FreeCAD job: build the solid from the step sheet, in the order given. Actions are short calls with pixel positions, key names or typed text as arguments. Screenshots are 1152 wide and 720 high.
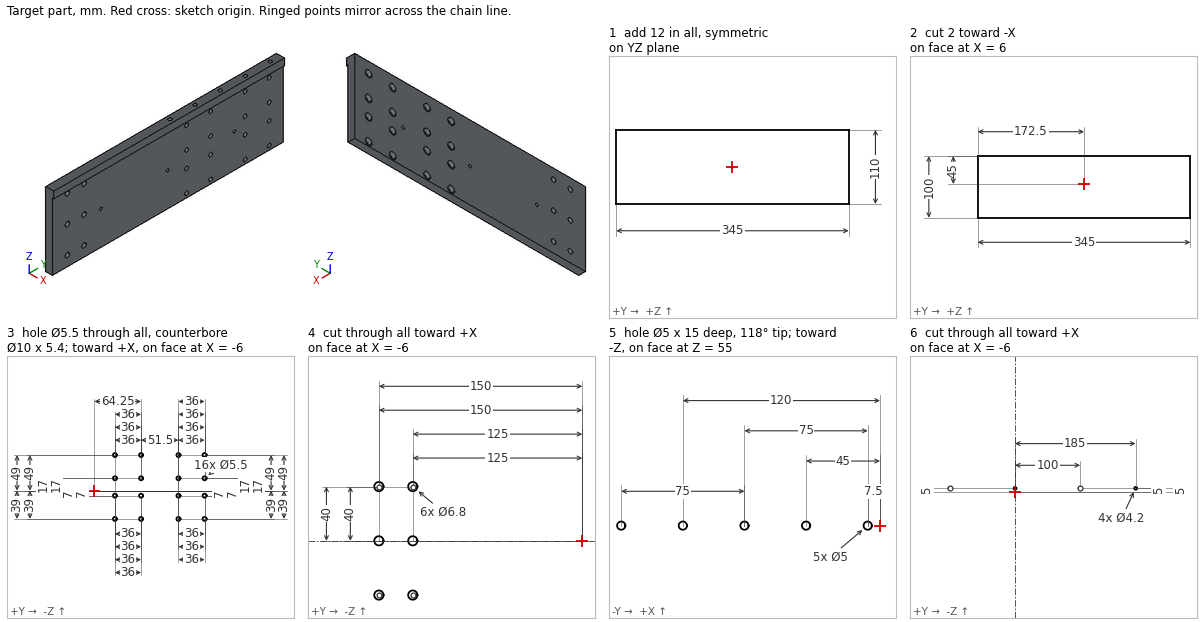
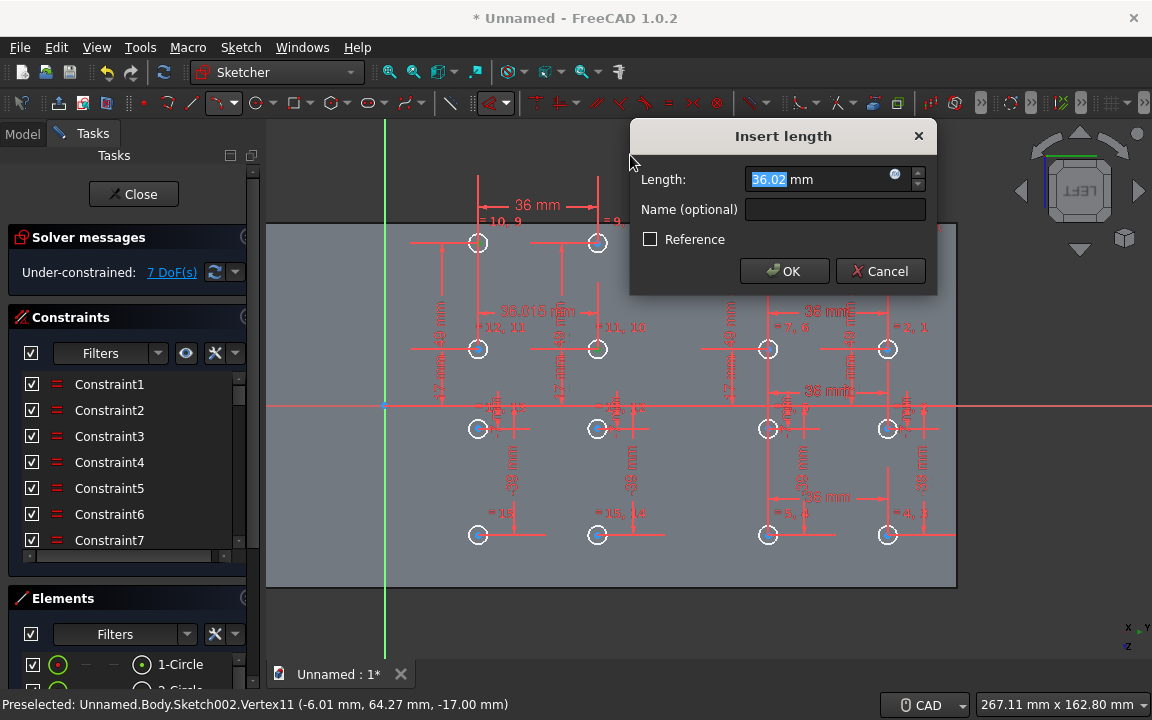
text(36)
key(Return)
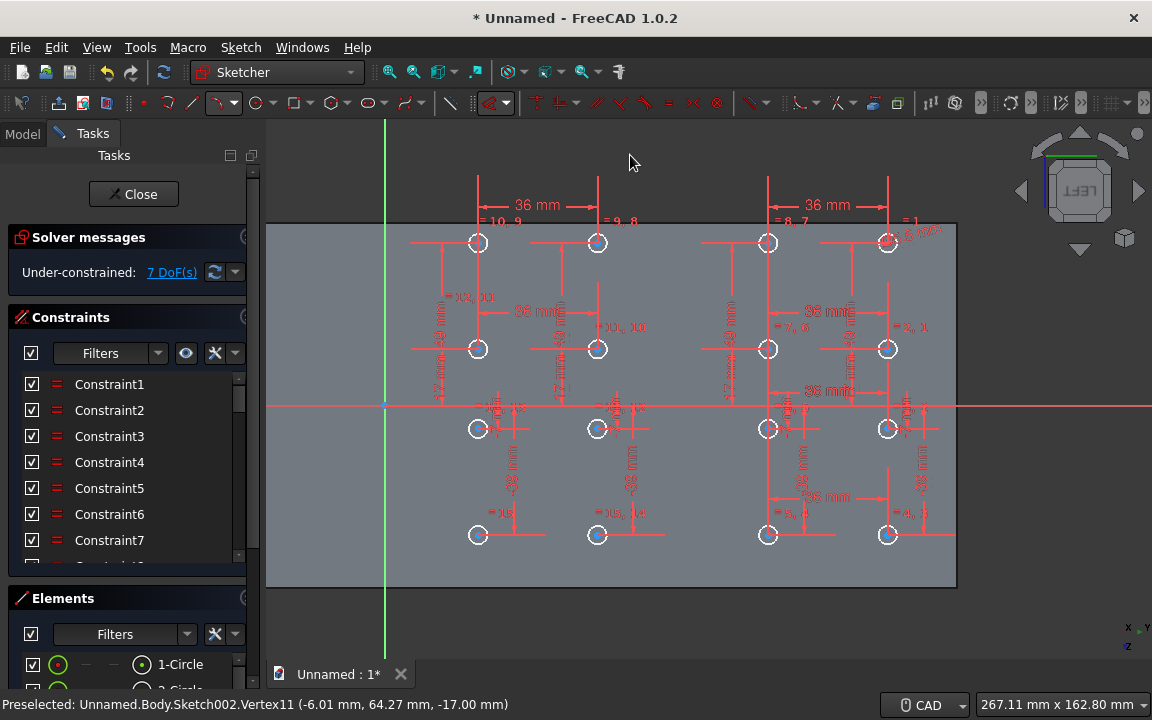
click(598, 349)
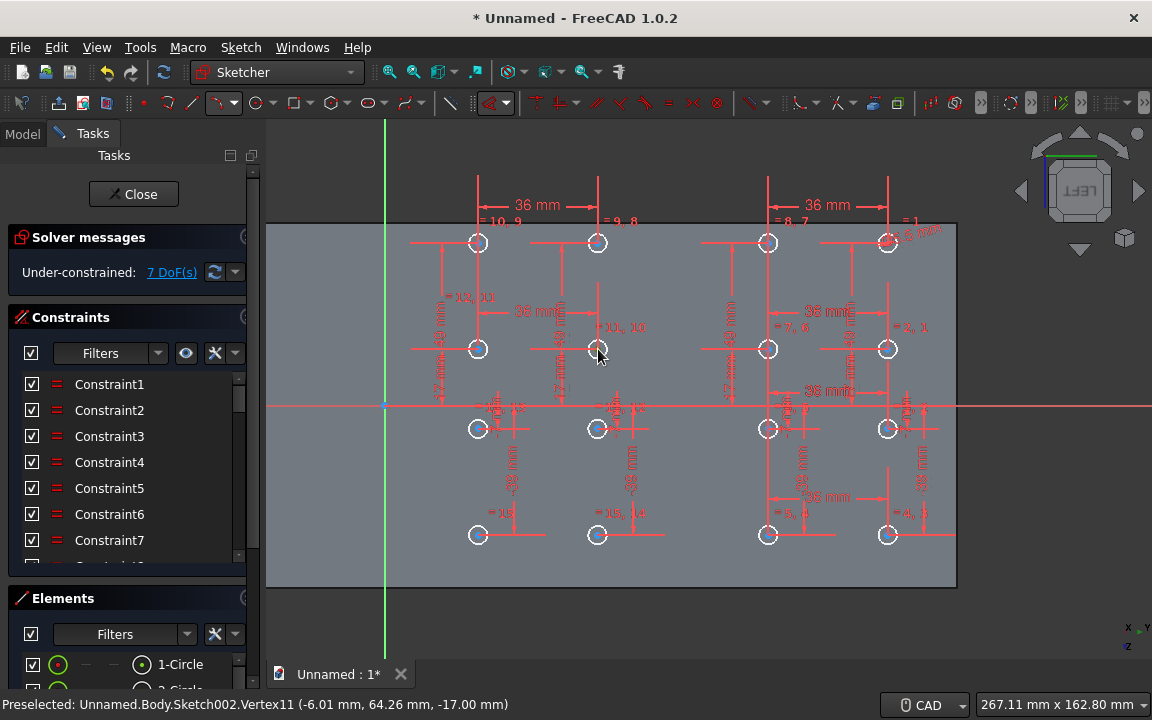
click(478, 349)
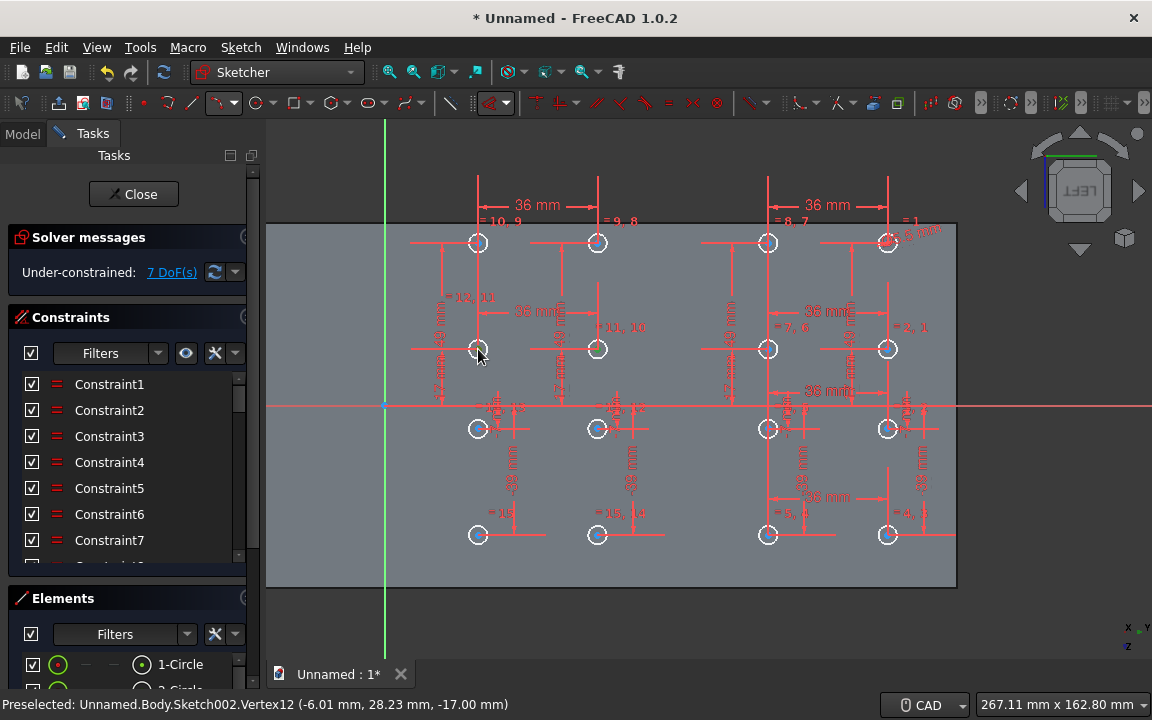
key(l)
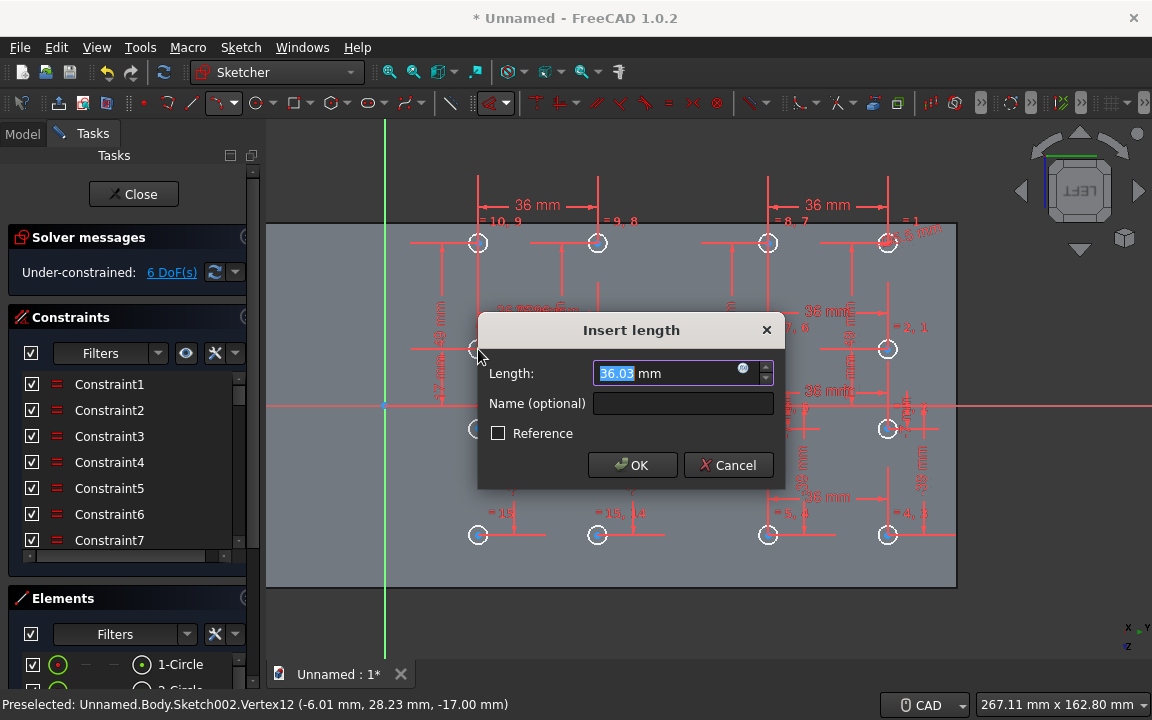
text(36)
key(Return)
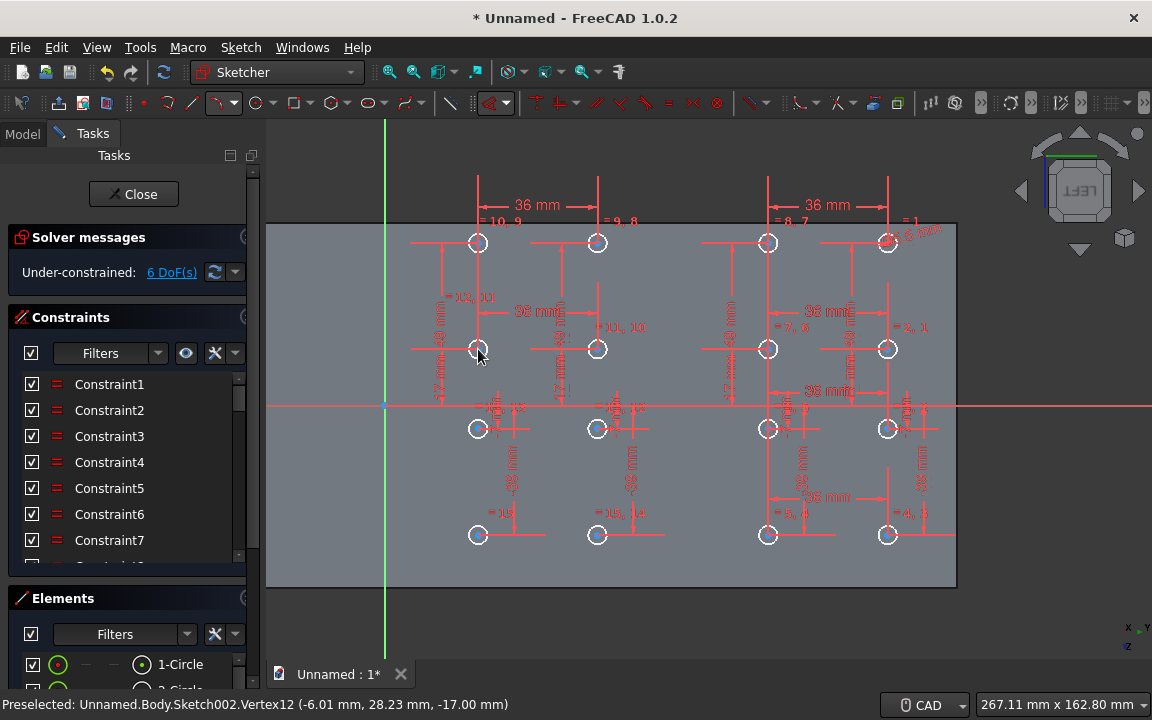
click(478, 349)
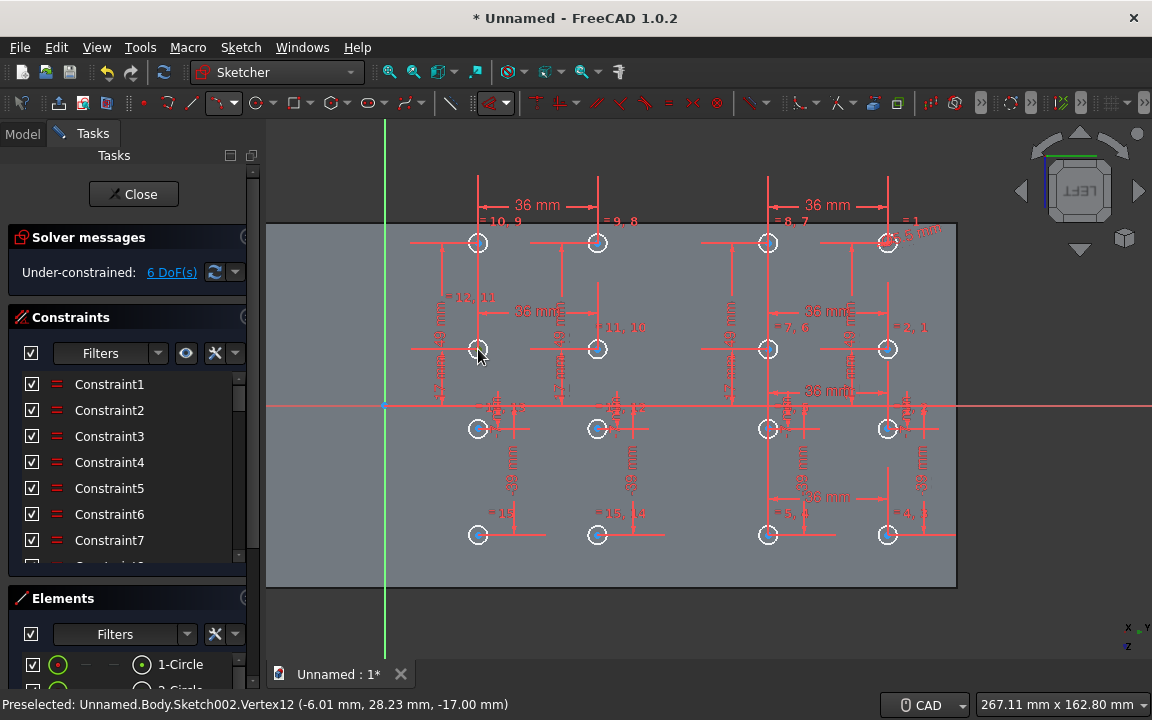
click(598, 429)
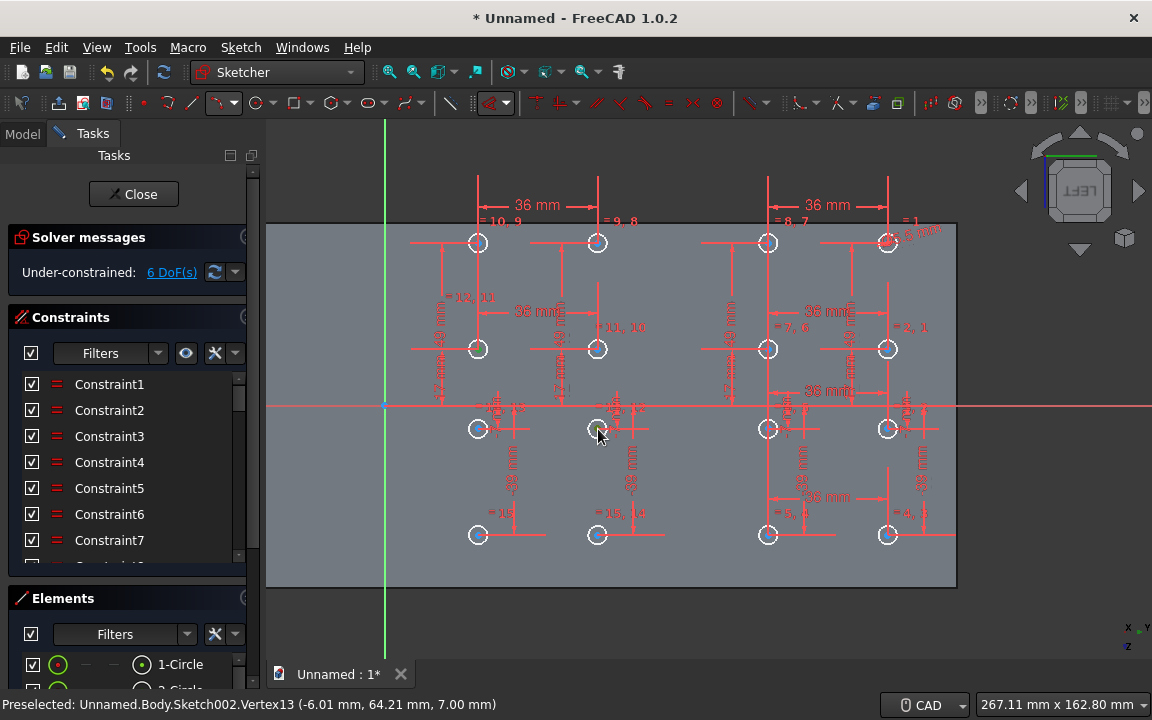
click(508, 104)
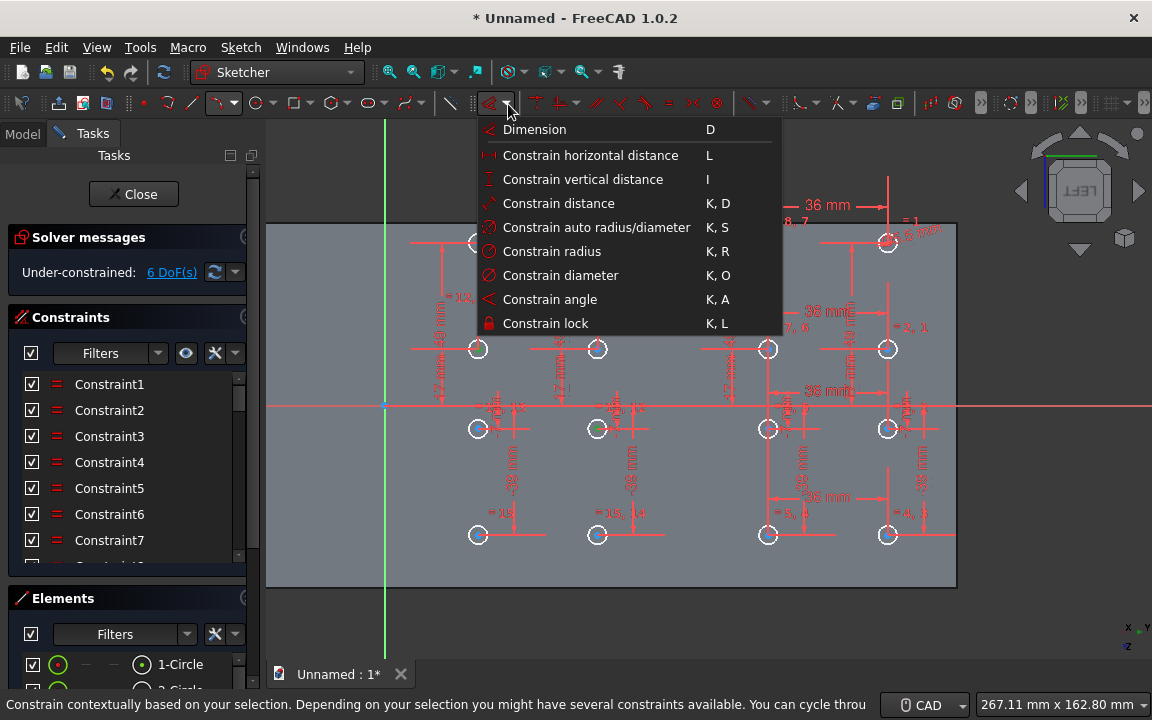
click(630, 155)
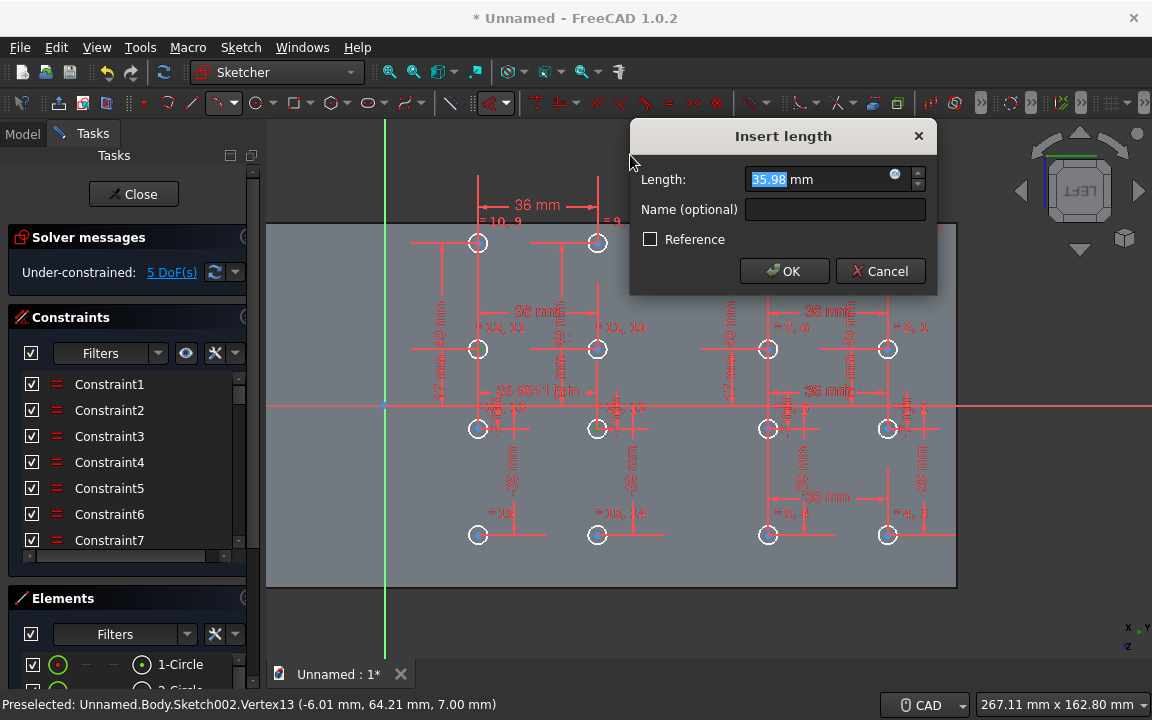
text(36)
key(Return)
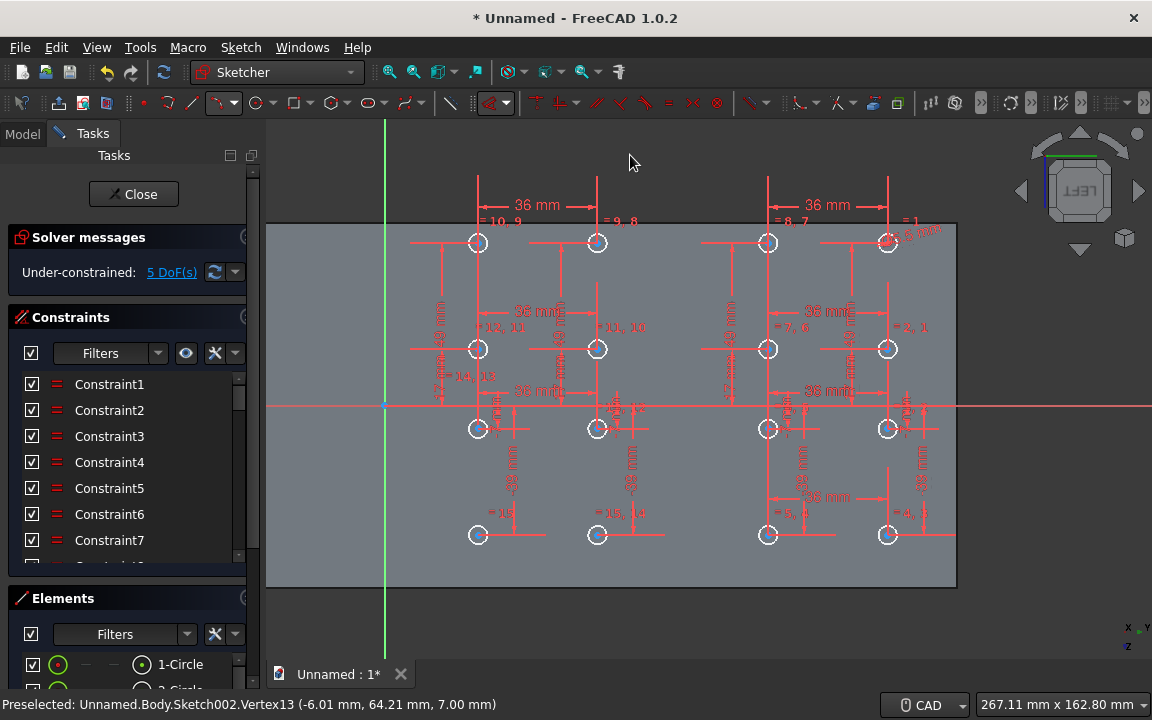
click(598, 429)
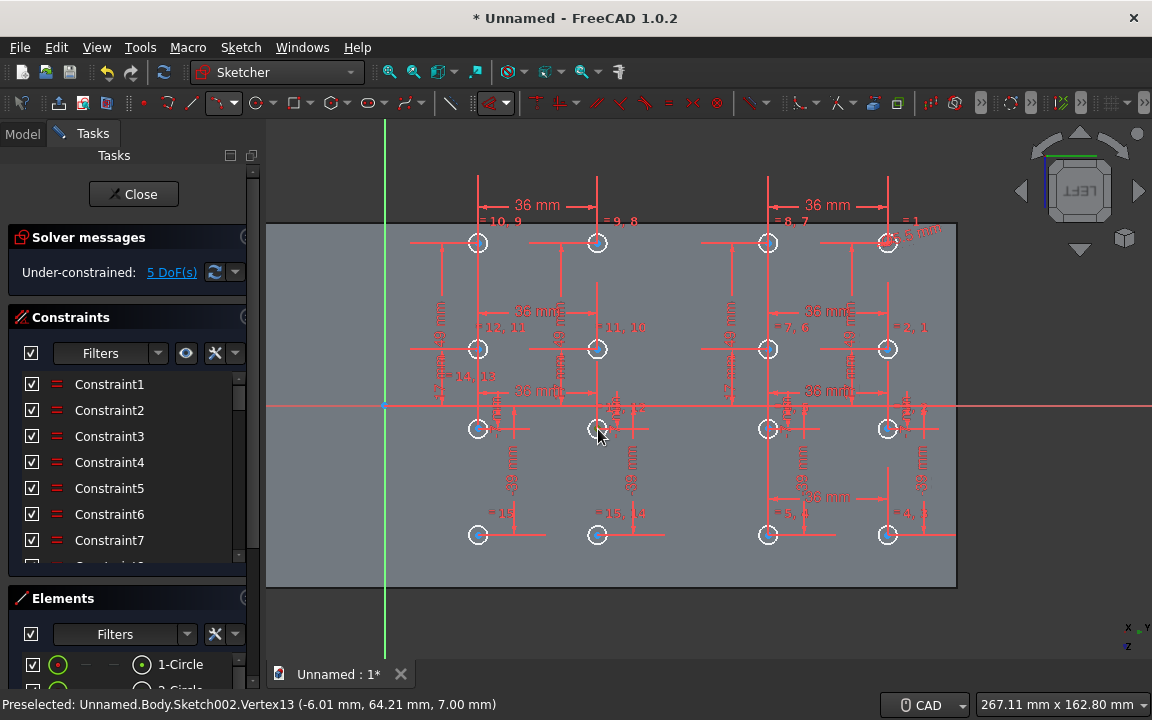
click(478, 429)